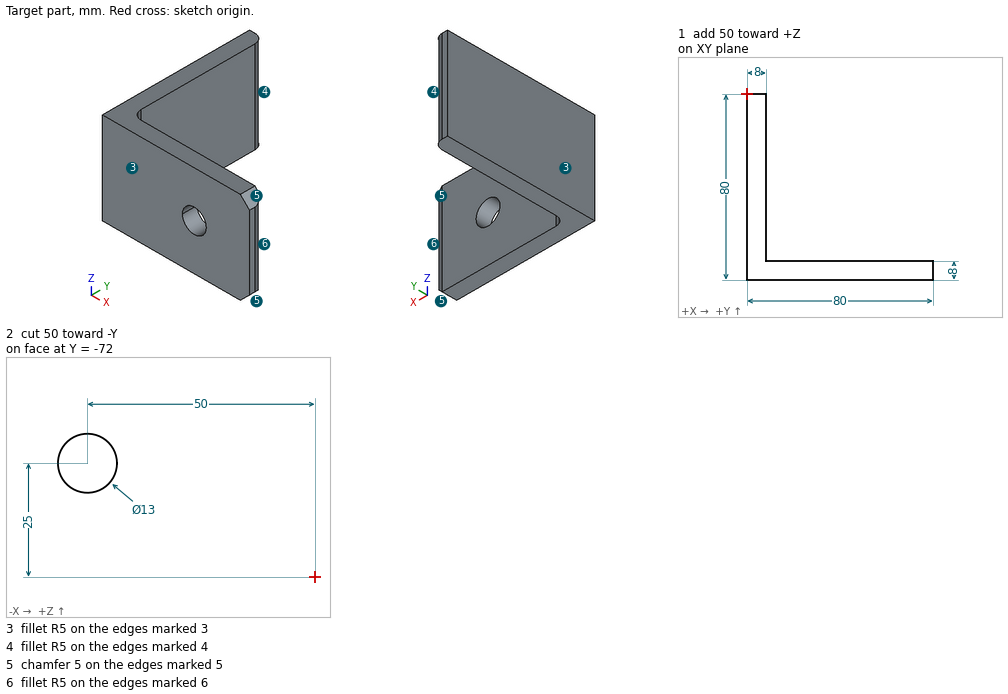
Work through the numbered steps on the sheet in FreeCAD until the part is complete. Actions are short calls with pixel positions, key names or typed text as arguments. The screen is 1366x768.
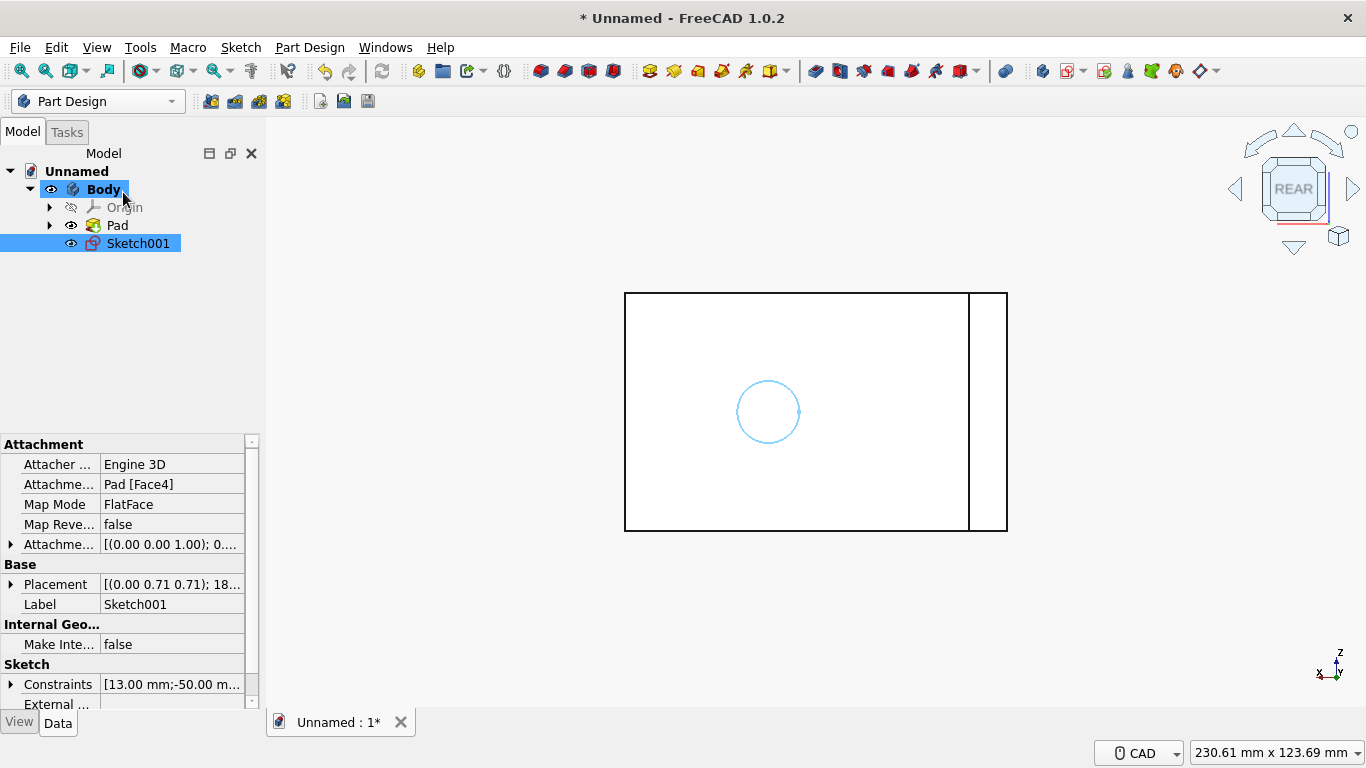
click(816, 72)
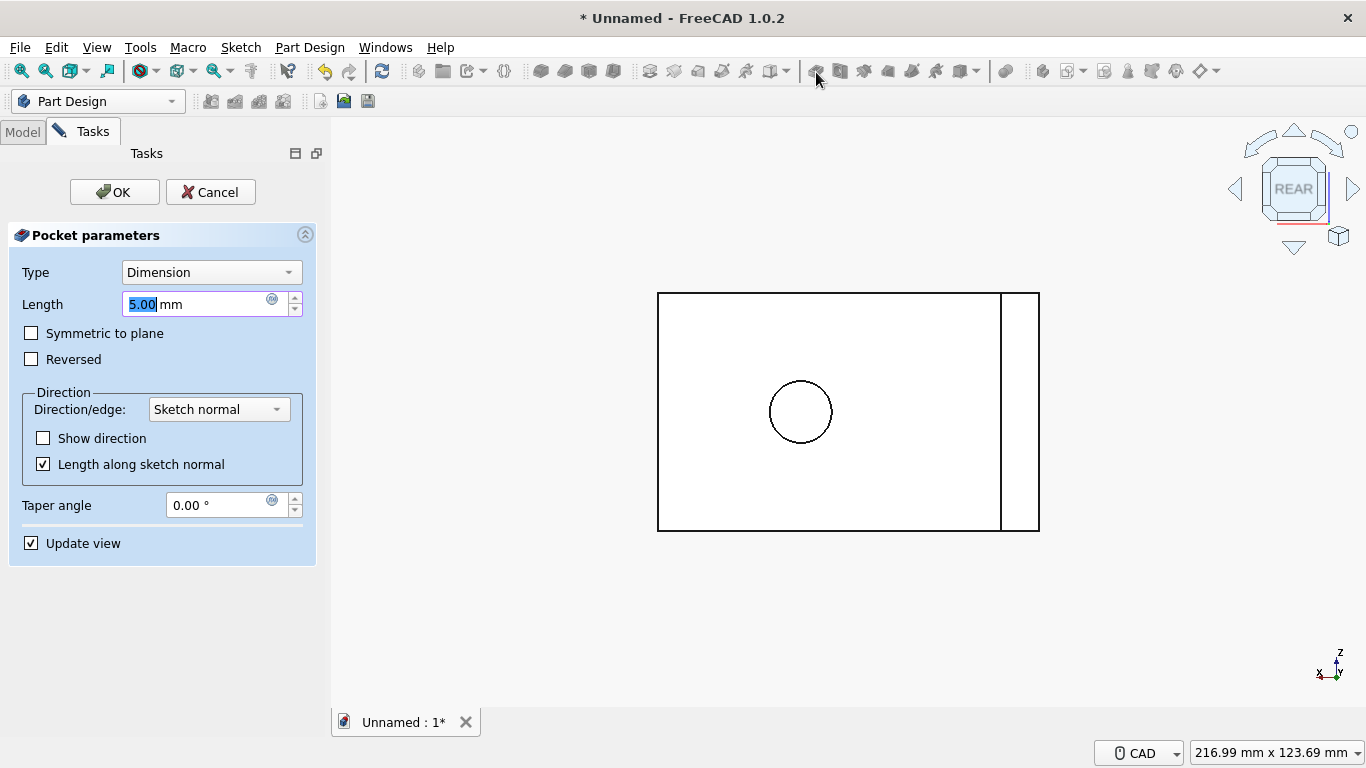
text(50)
key(Tab)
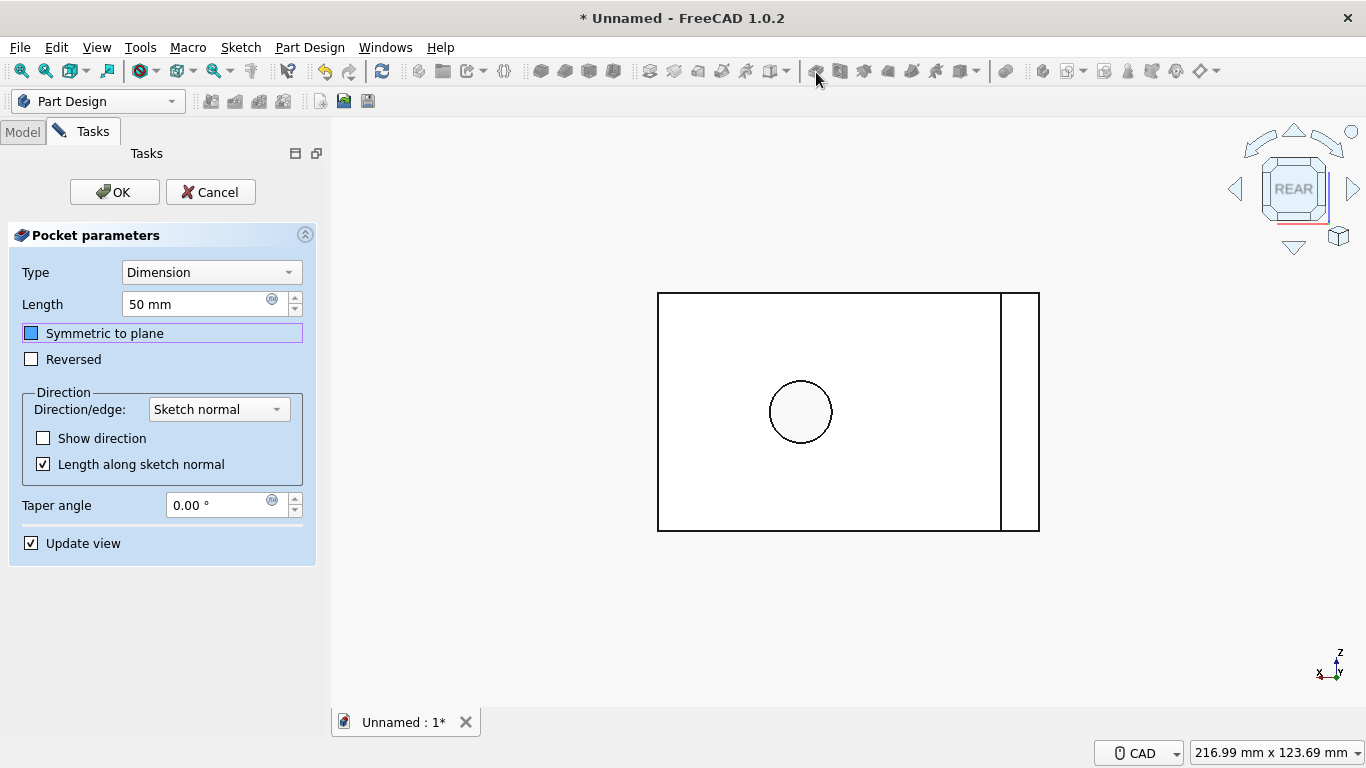
click(115, 192)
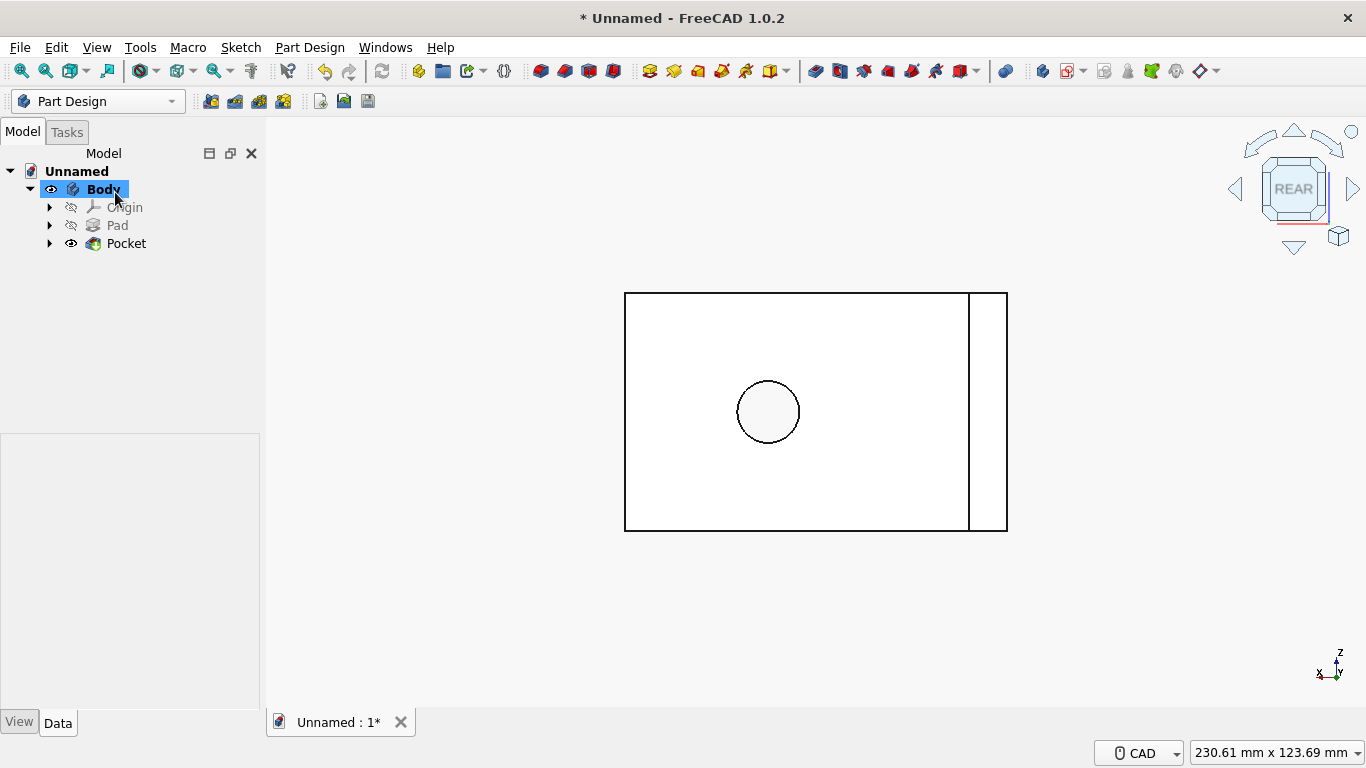
click(22, 72)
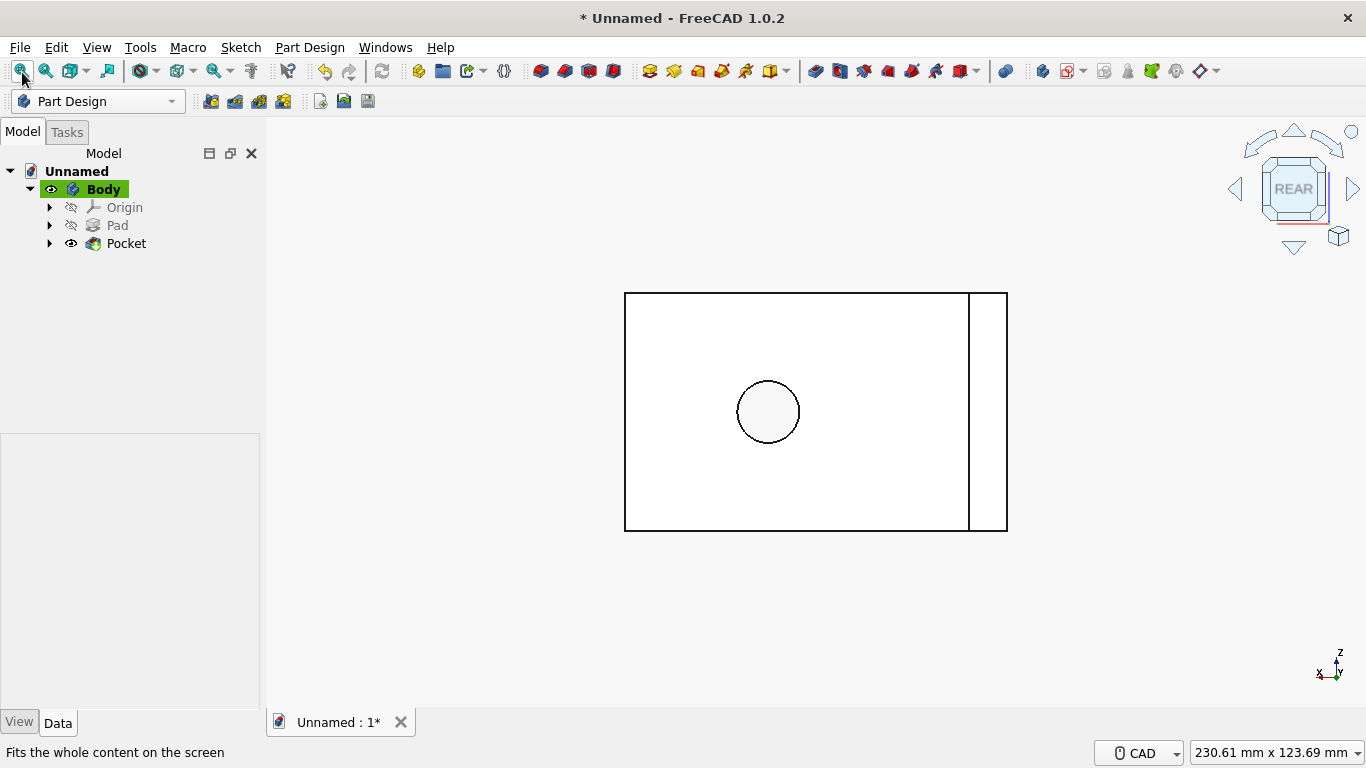
key(0)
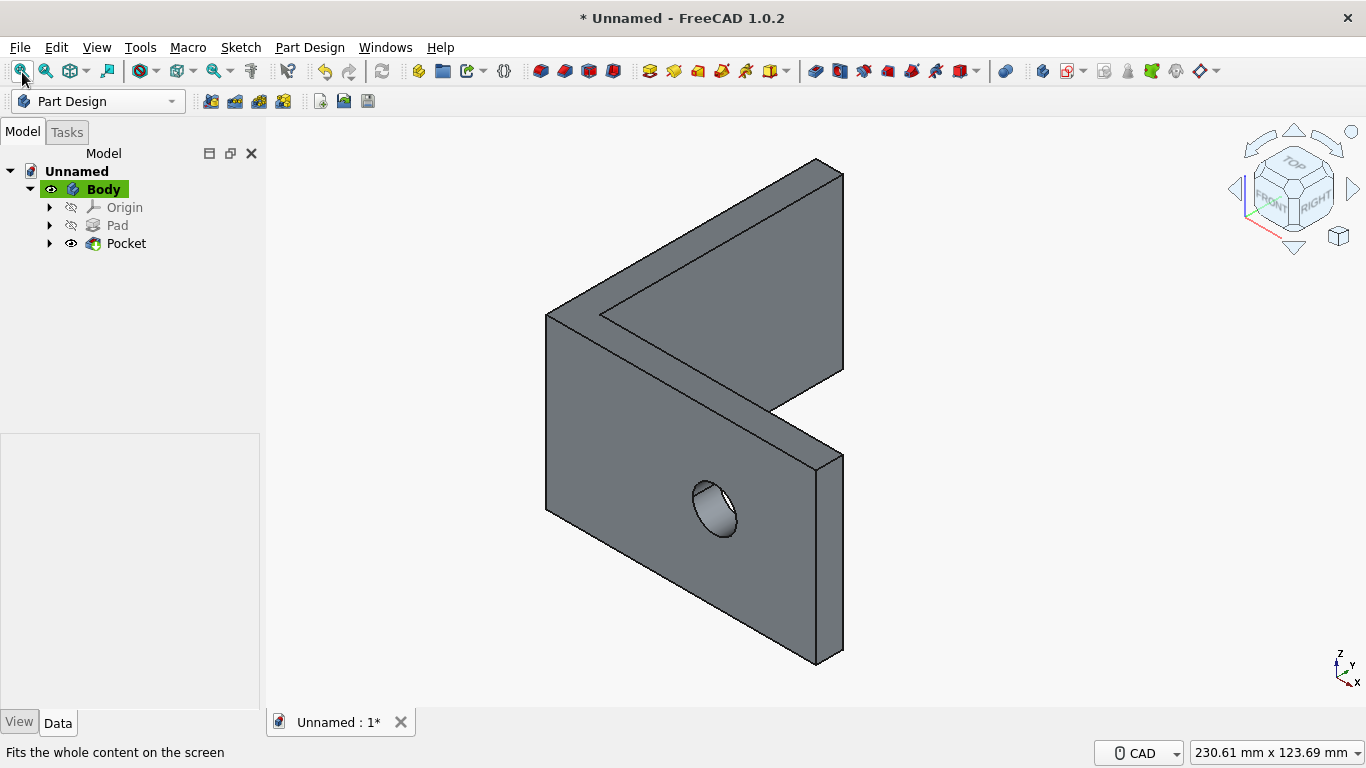
key(2)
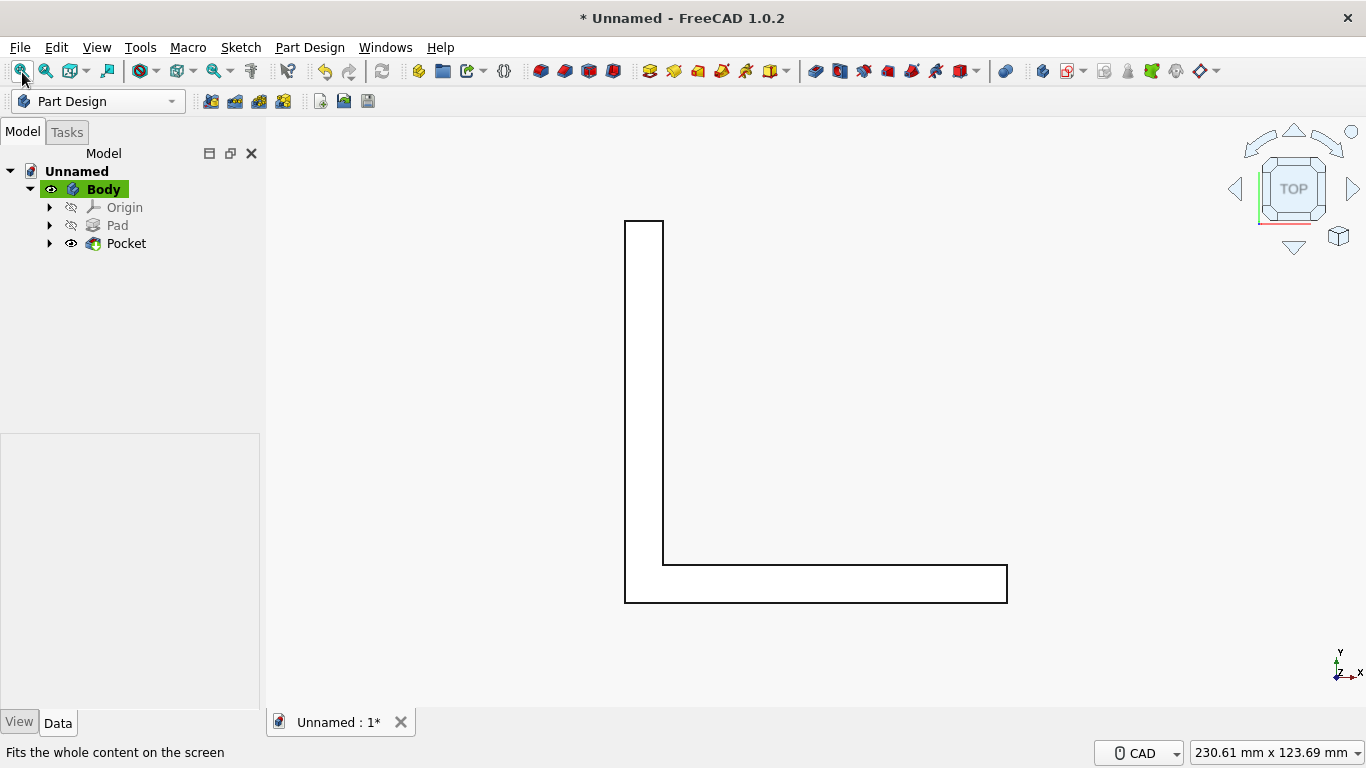
key(1)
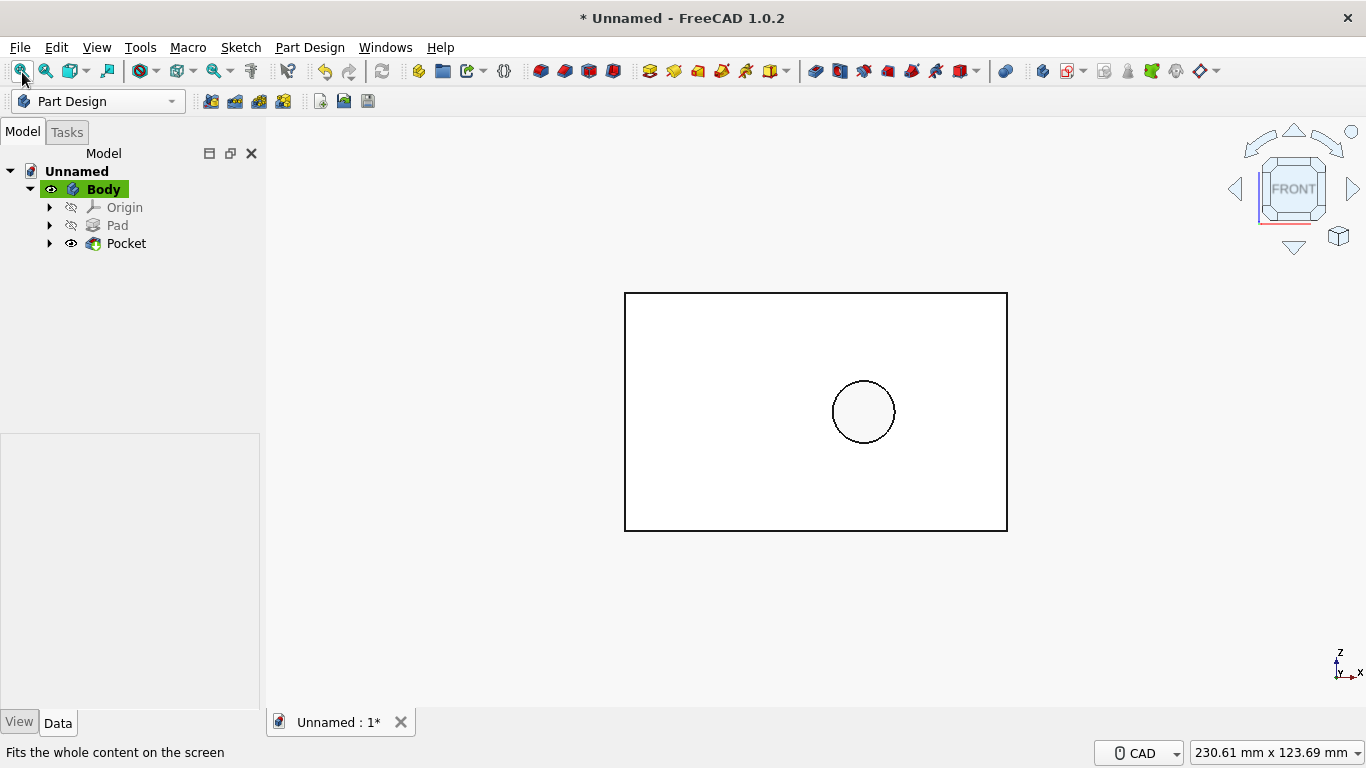
click(22, 72)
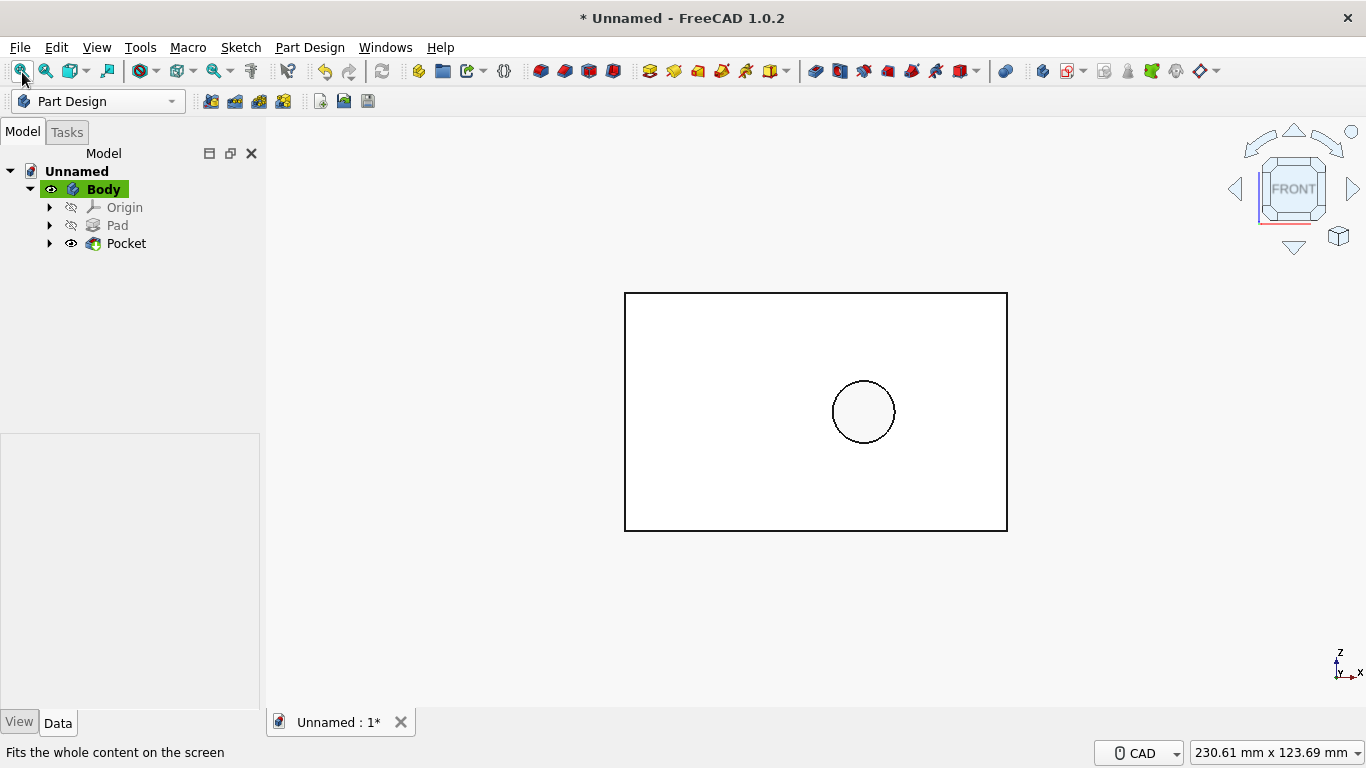
key(3)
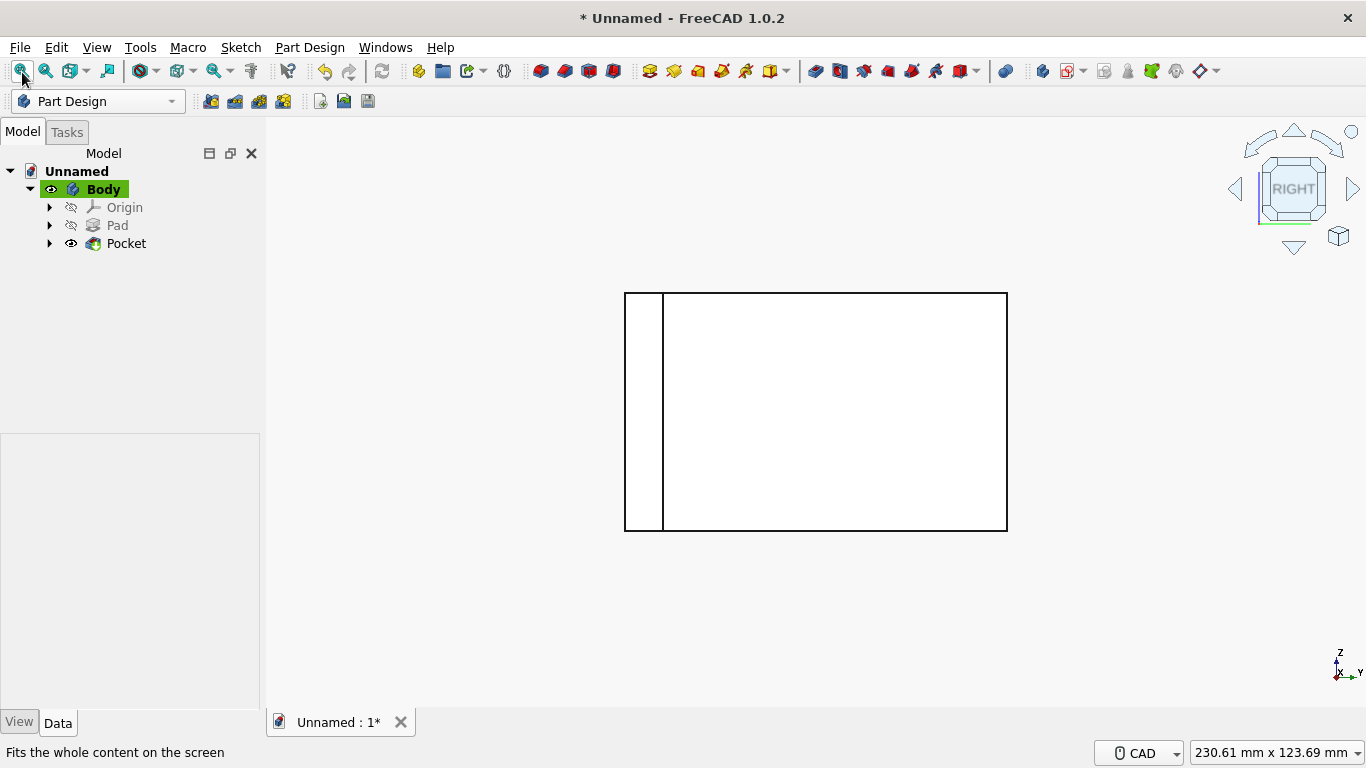
click(22, 72)